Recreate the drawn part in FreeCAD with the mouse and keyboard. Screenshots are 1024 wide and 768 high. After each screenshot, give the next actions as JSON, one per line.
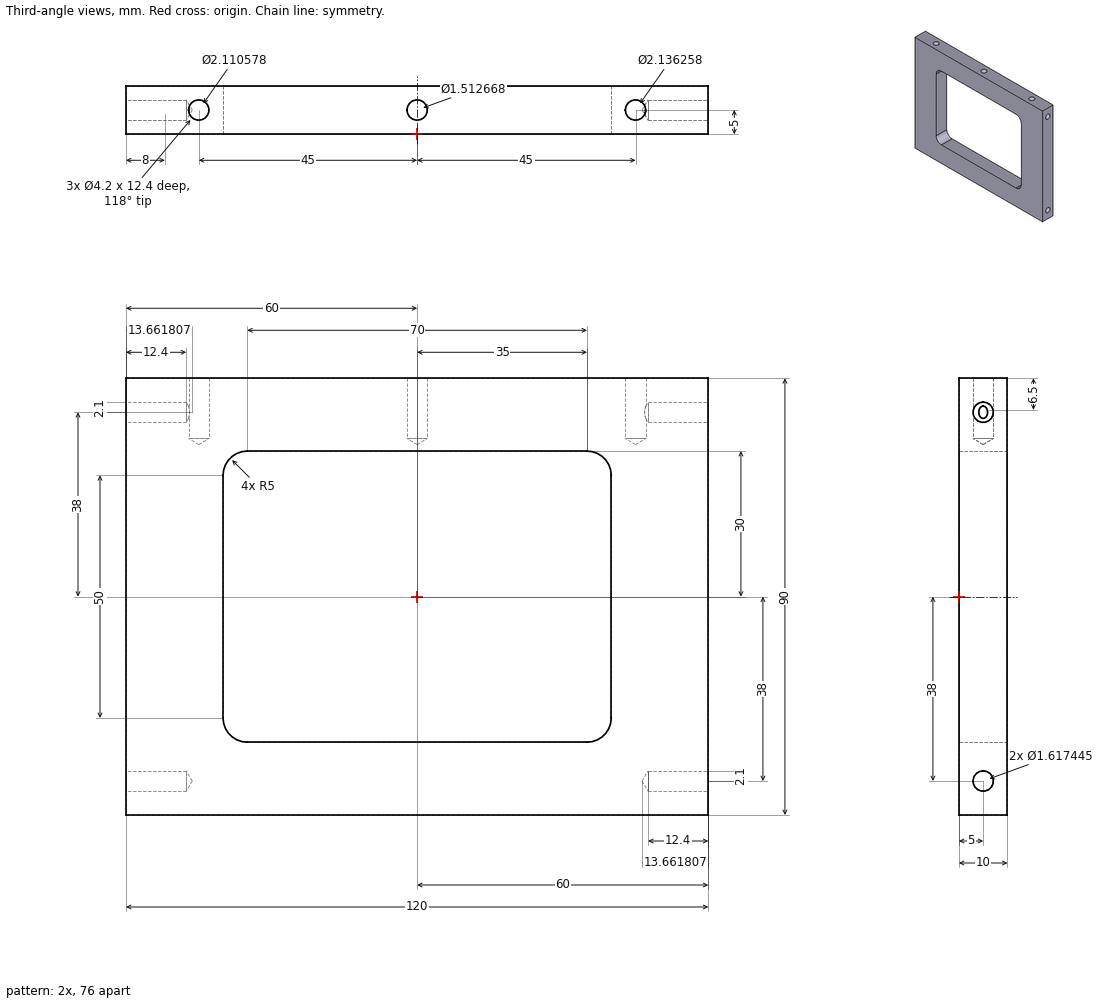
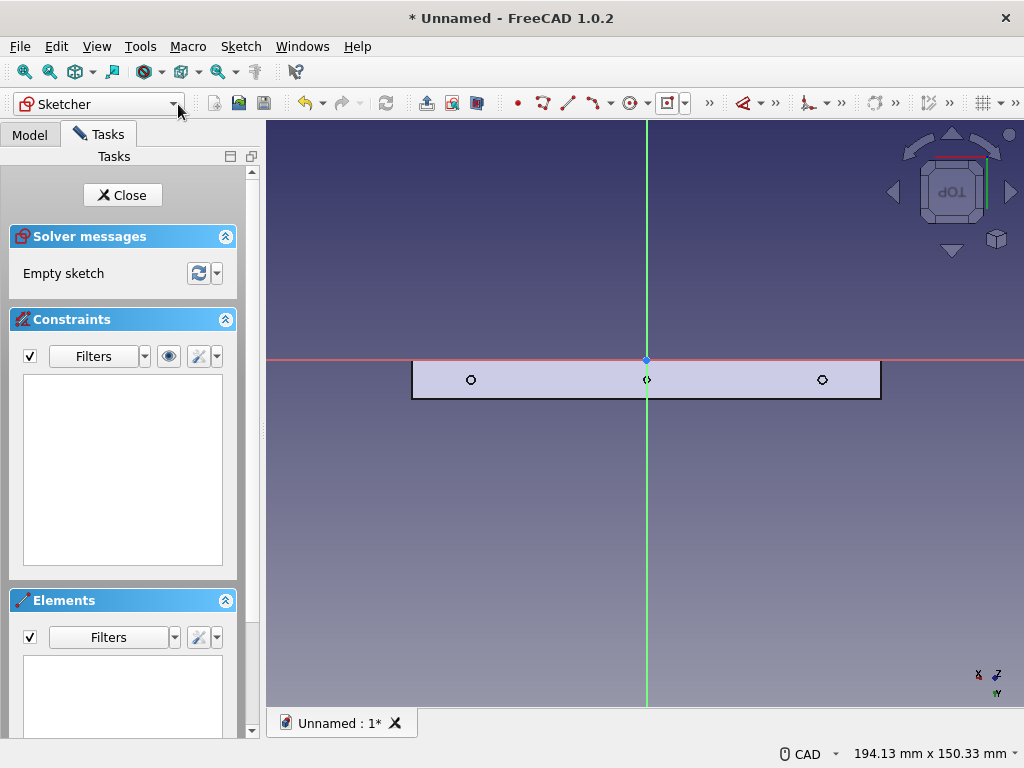
{"action": "left_click", "coordinate": [630, 104]}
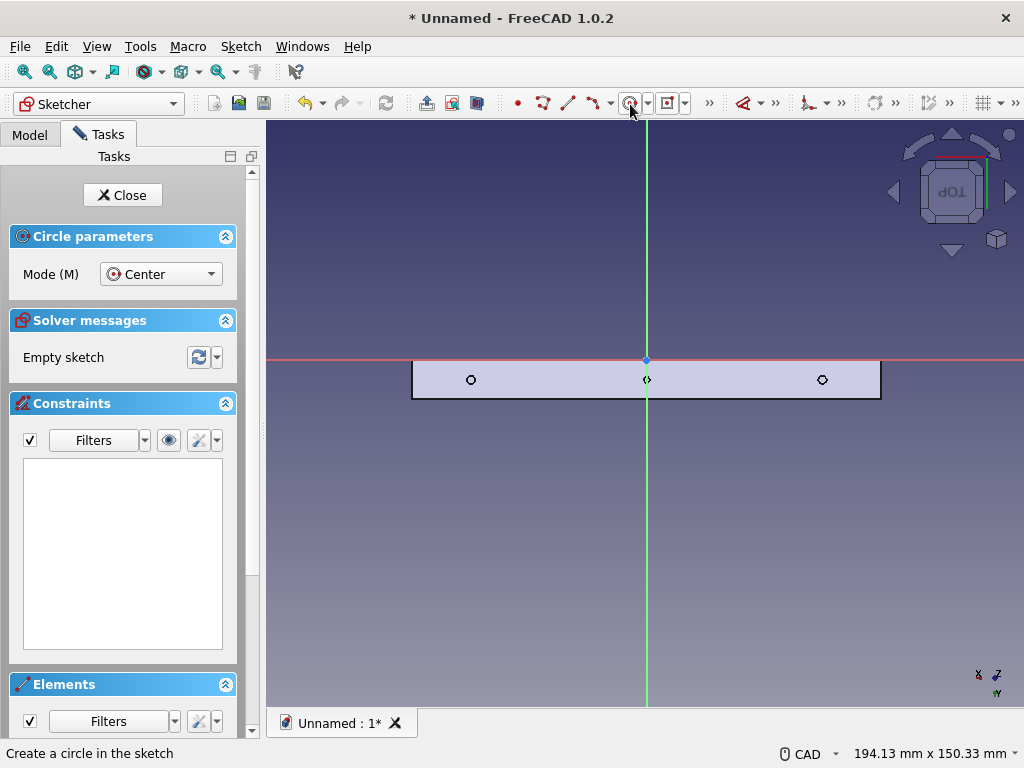
{"action": "scroll", "coordinate": [822, 380], "scroll_direction": "up", "scroll_amount": 6}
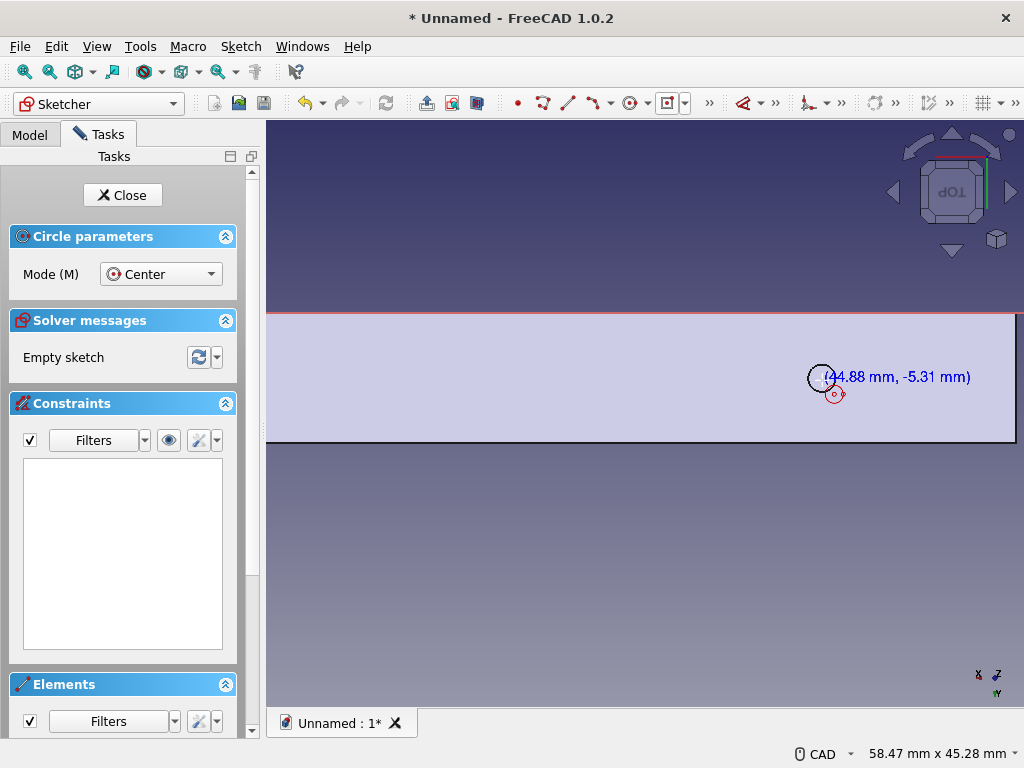
{"action": "left_click", "coordinate": [822, 378]}
{"action": "mouse_move", "coordinate": [841, 359]}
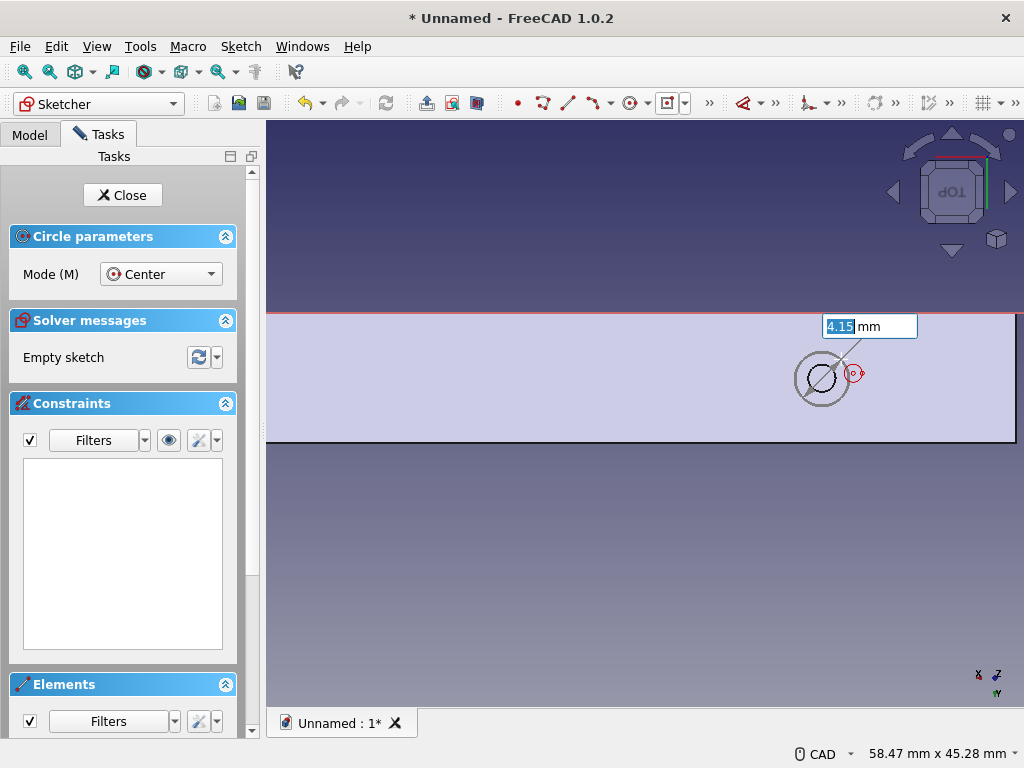
{"action": "type", "text": "4.2"}
{"action": "key", "text": "Return"}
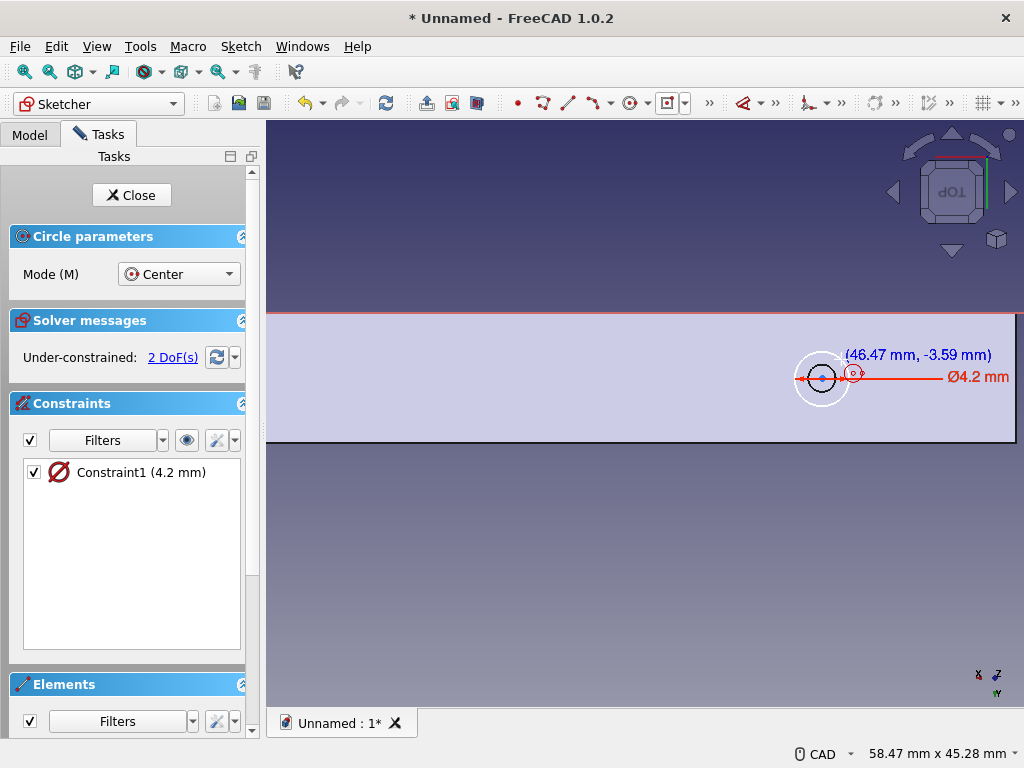
{"action": "scroll", "coordinate": [722, 437], "scroll_direction": "down", "scroll_amount": 6}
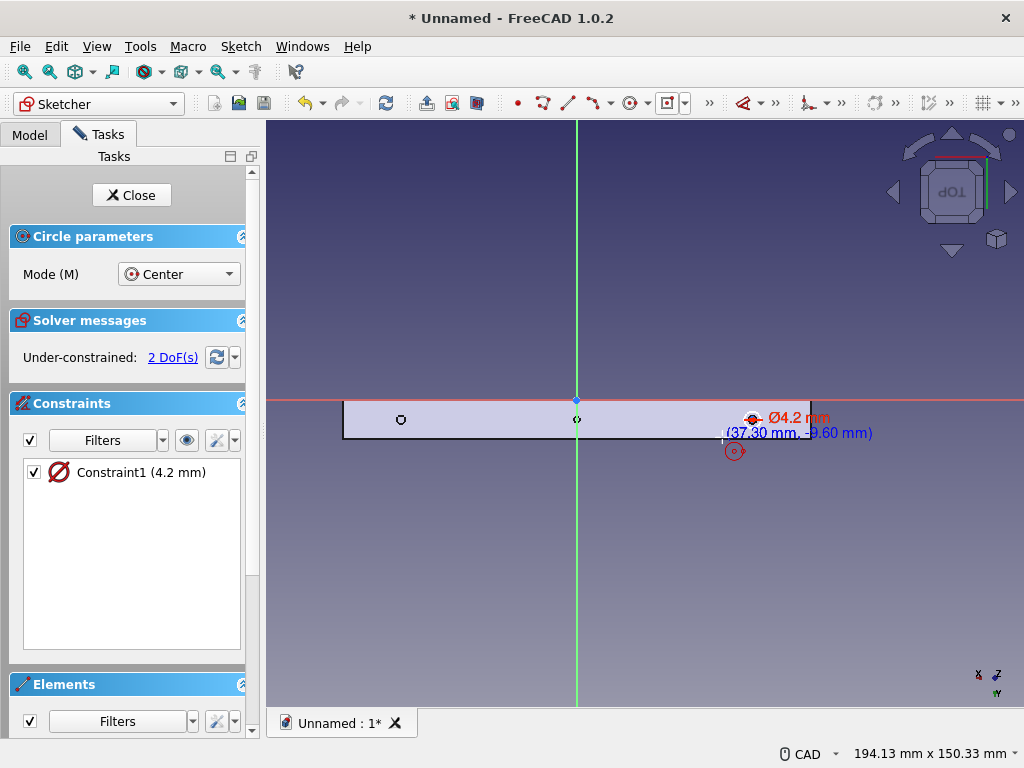
{"action": "scroll", "coordinate": [577, 420], "scroll_direction": "up", "scroll_amount": 6}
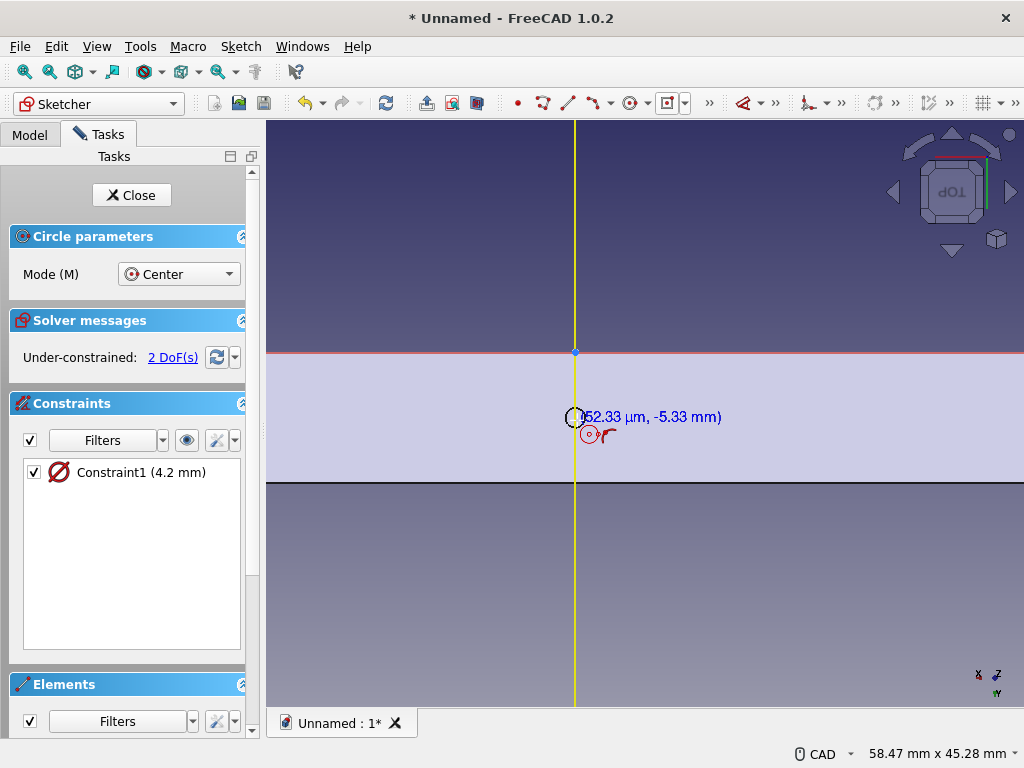
{"action": "left_click", "coordinate": [575, 418]}
{"action": "mouse_move", "coordinate": [595, 399]}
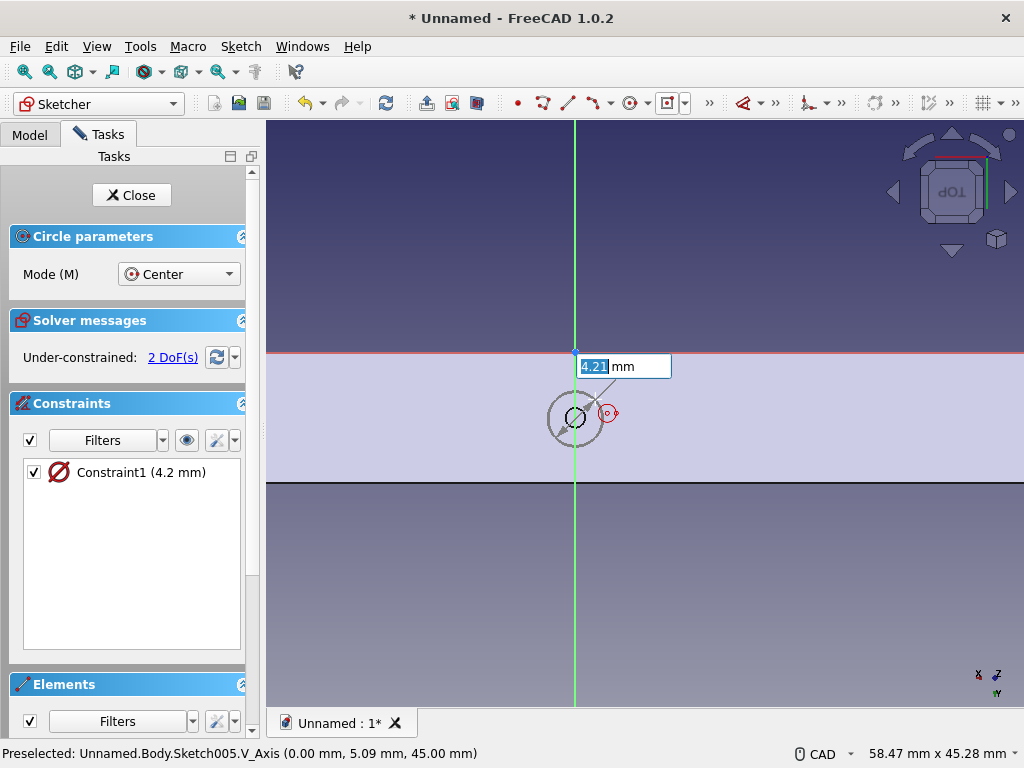
{"action": "type", "text": "4.2"}
{"action": "key", "text": "Return"}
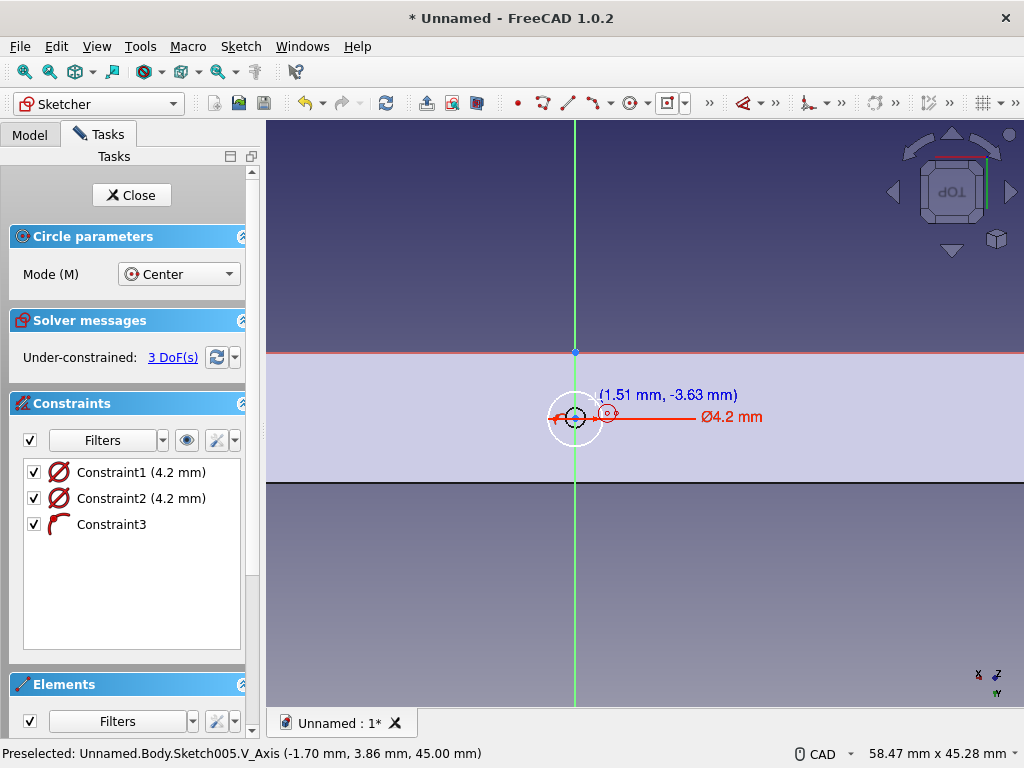
{"action": "scroll", "coordinate": [577, 420], "scroll_direction": "down", "scroll_amount": 6}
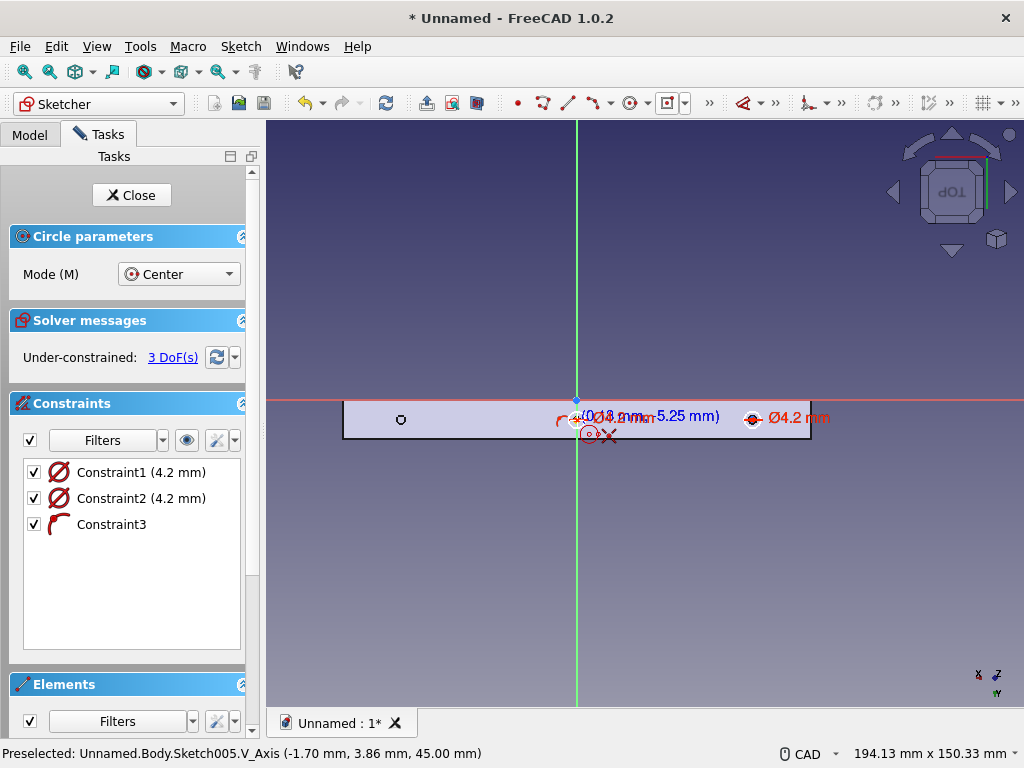
{"action": "scroll", "coordinate": [401, 420], "scroll_direction": "up", "scroll_amount": 6}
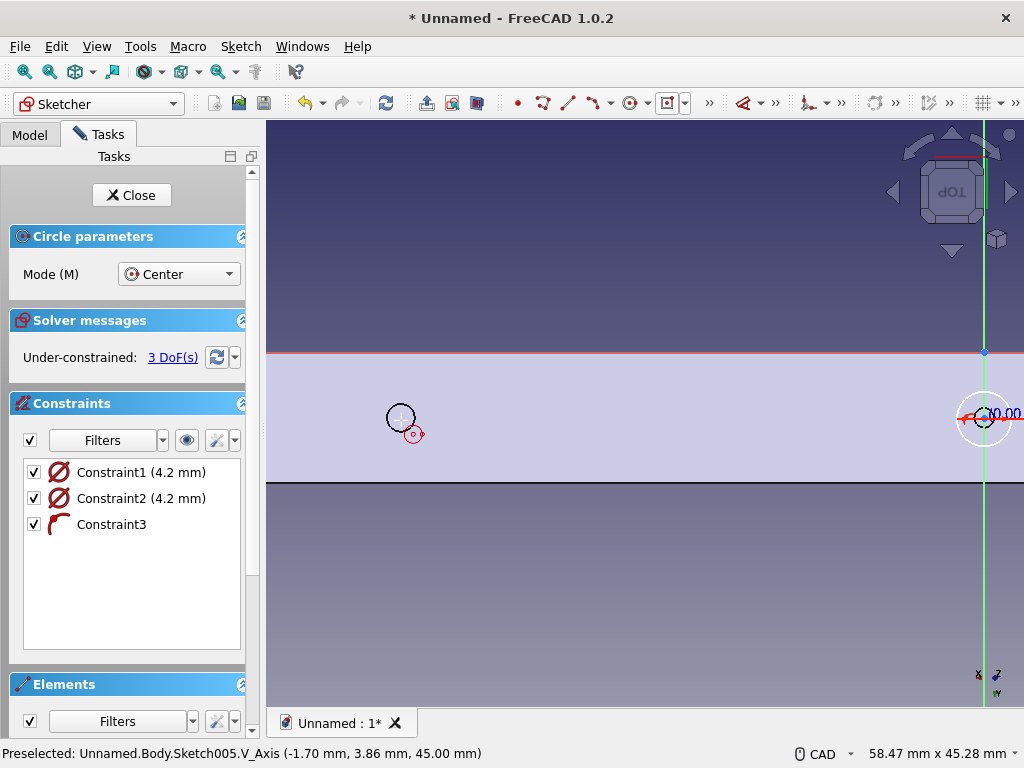
{"action": "left_click", "coordinate": [401, 418]}
{"action": "mouse_move", "coordinate": [420, 399]}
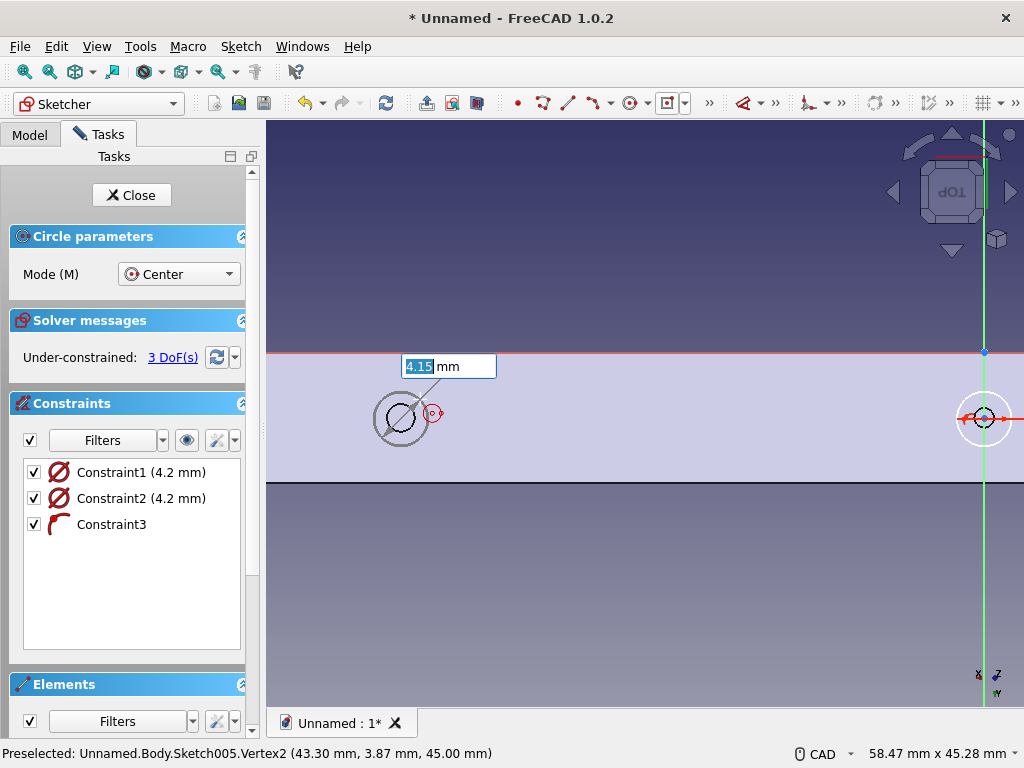
{"action": "type", "text": "4.2"}
{"action": "key", "text": "Return"}
{"action": "key", "text": "Escape"}